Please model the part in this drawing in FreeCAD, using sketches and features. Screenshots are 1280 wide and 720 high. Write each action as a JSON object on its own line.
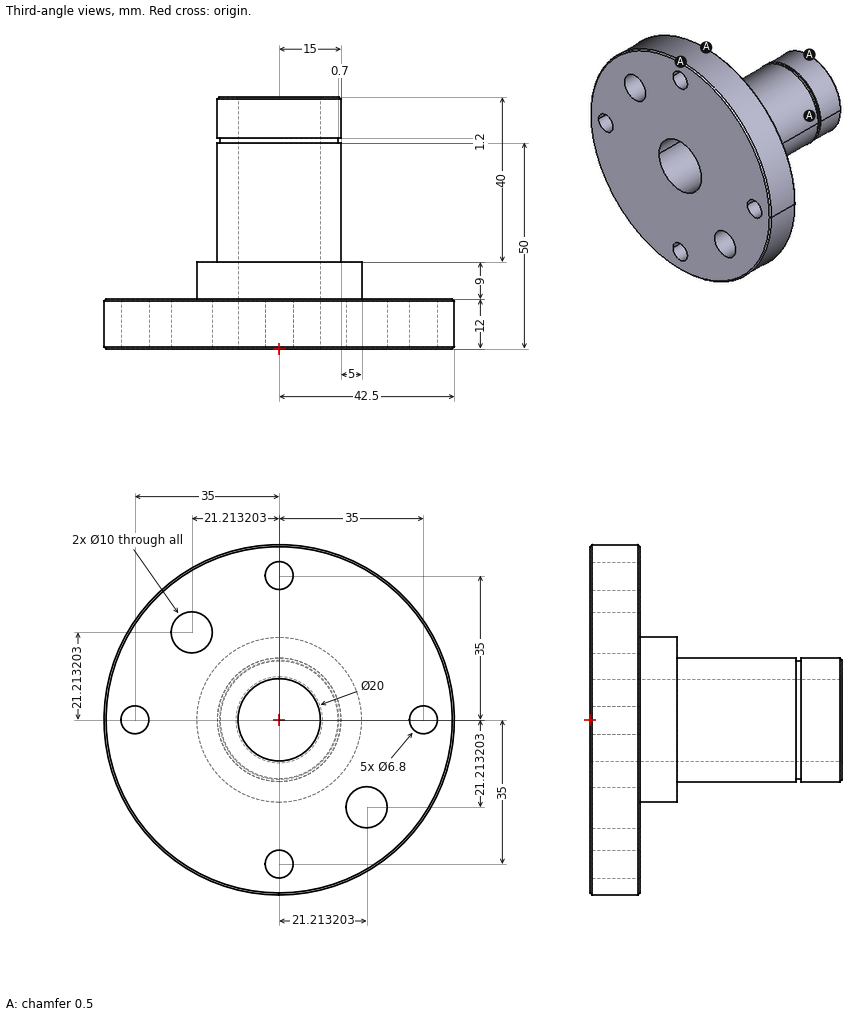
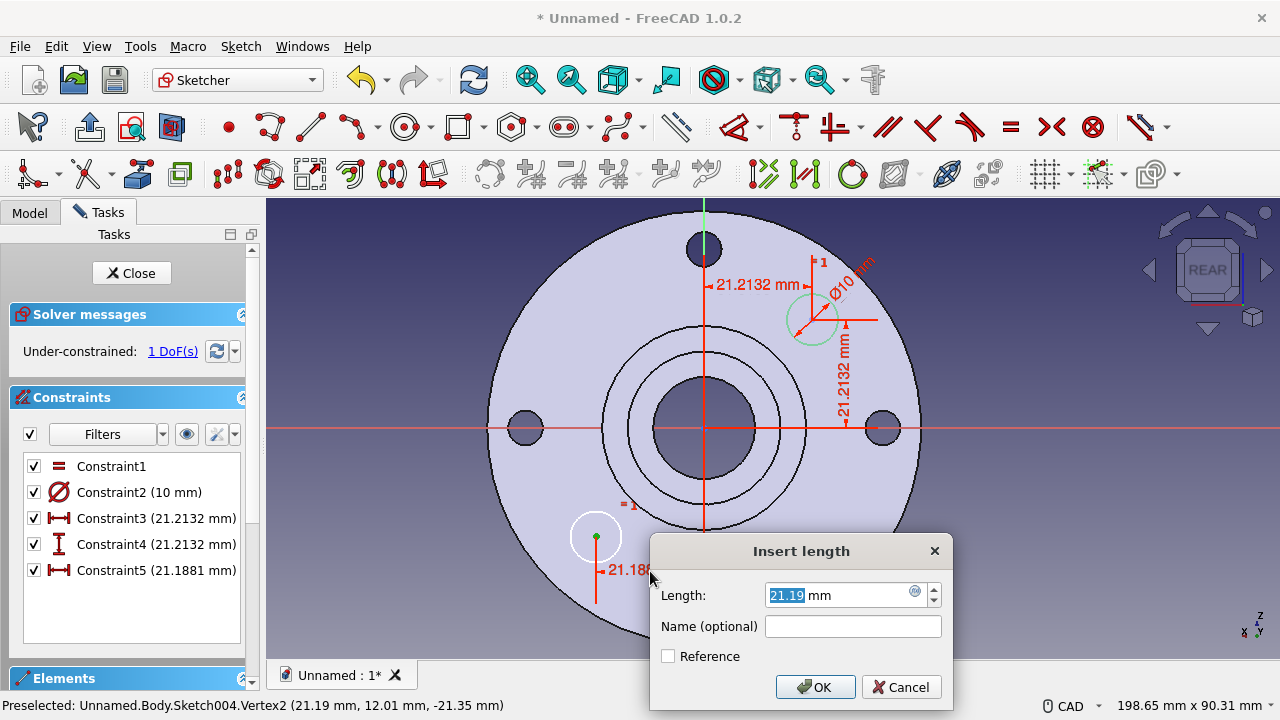
{"action": "type", "text": "21.213203"}
{"action": "key", "text": "Return"}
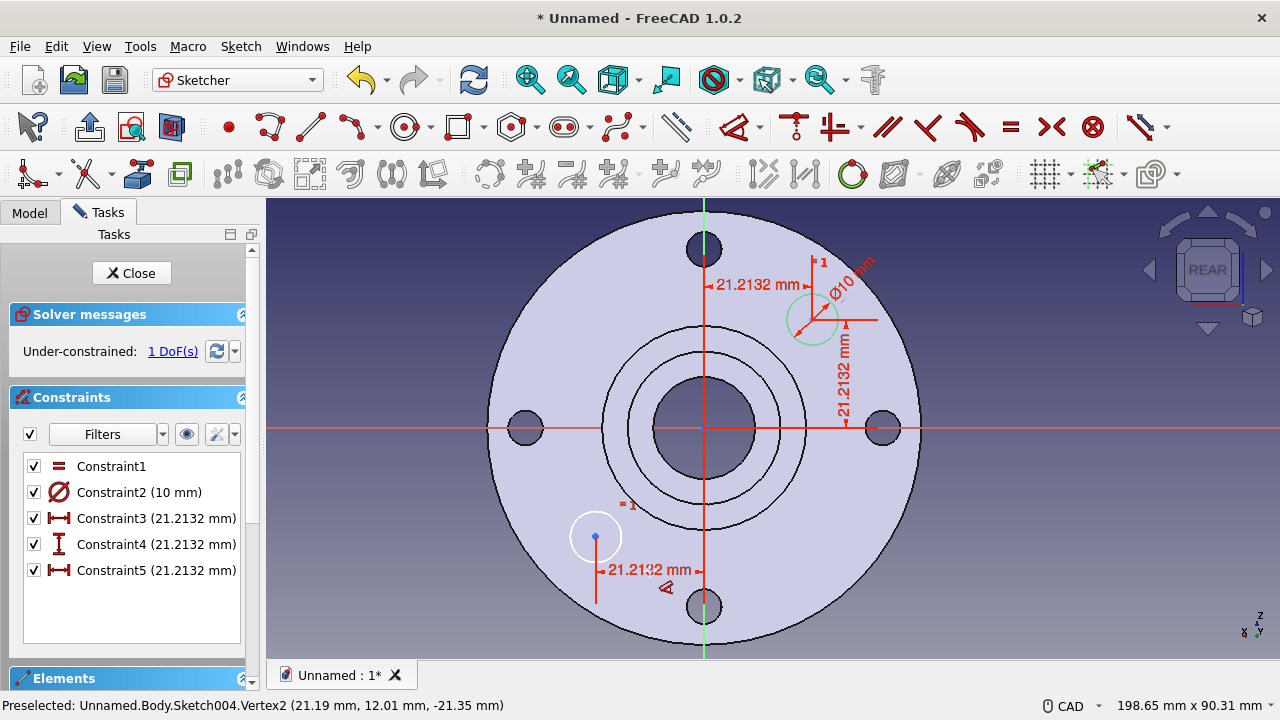
{"action": "left_click", "coordinate": [596, 537]}
{"action": "left_click", "coordinate": [562, 483]}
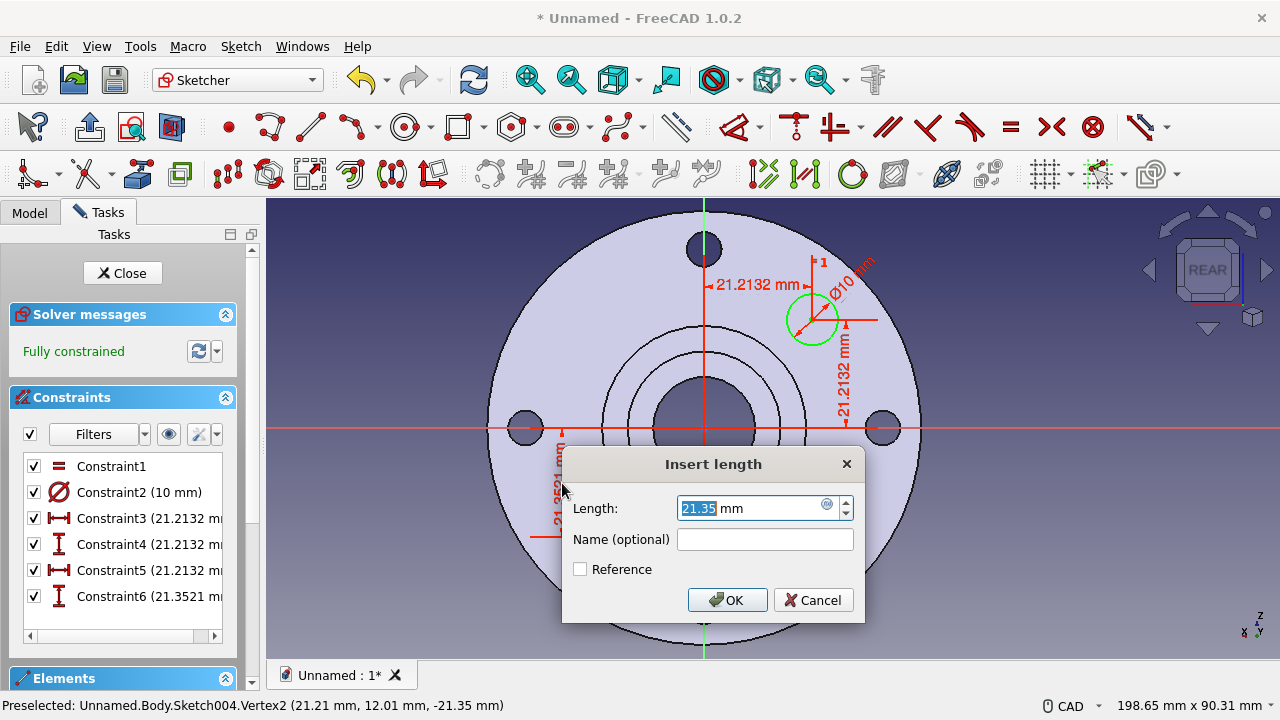
{"action": "type", "text": "21.213203"}
{"action": "key", "text": "Return"}
{"action": "key", "text": "Escape"}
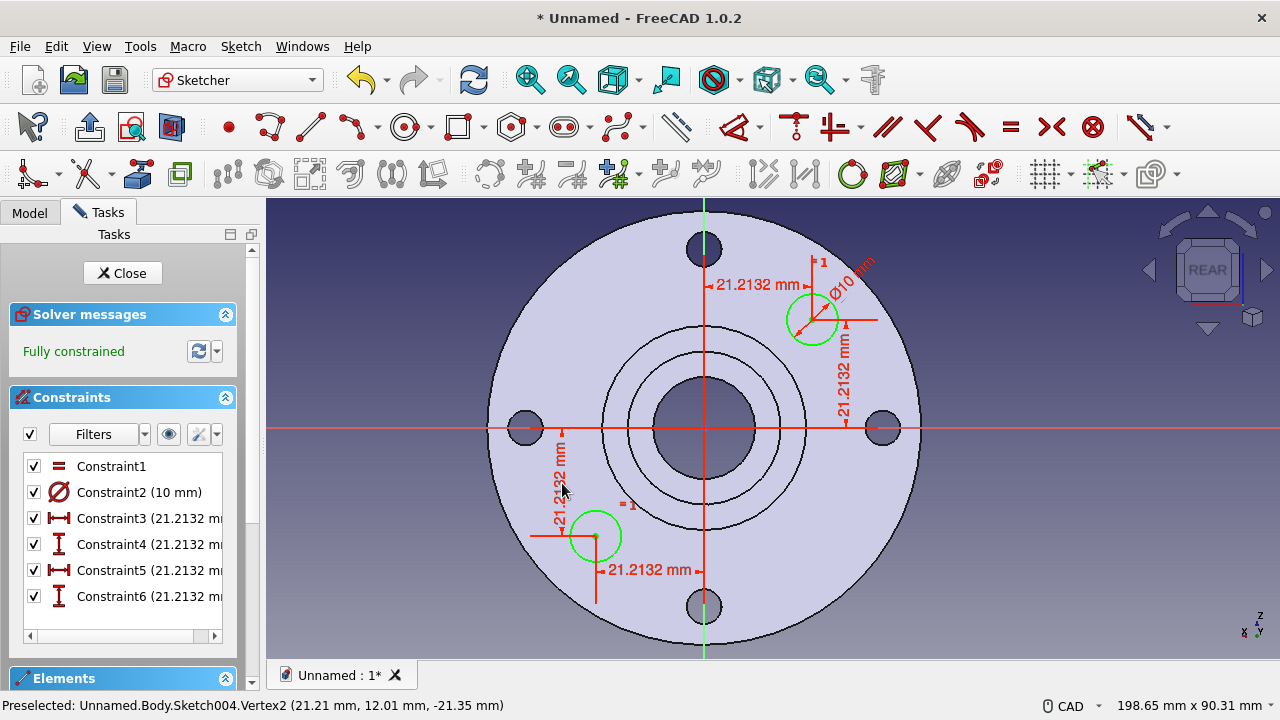
{"action": "left_click", "coordinate": [123, 273]}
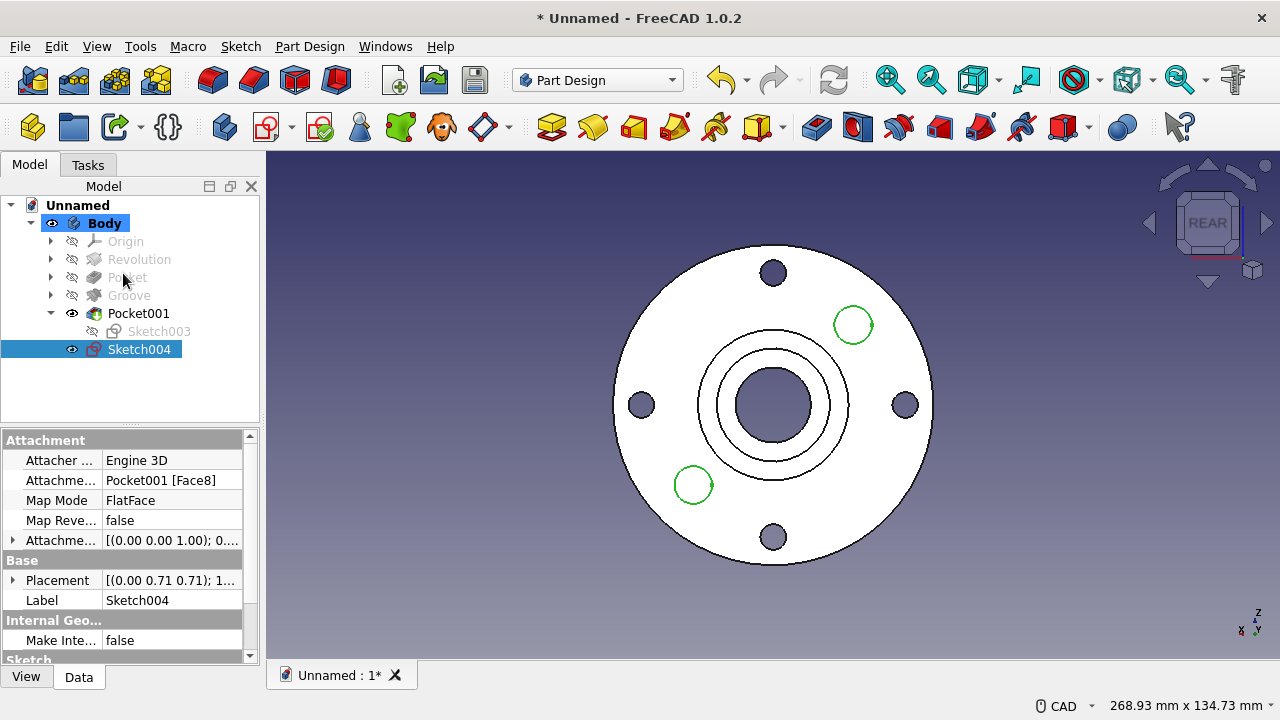
{"action": "left_click", "coordinate": [858, 128]}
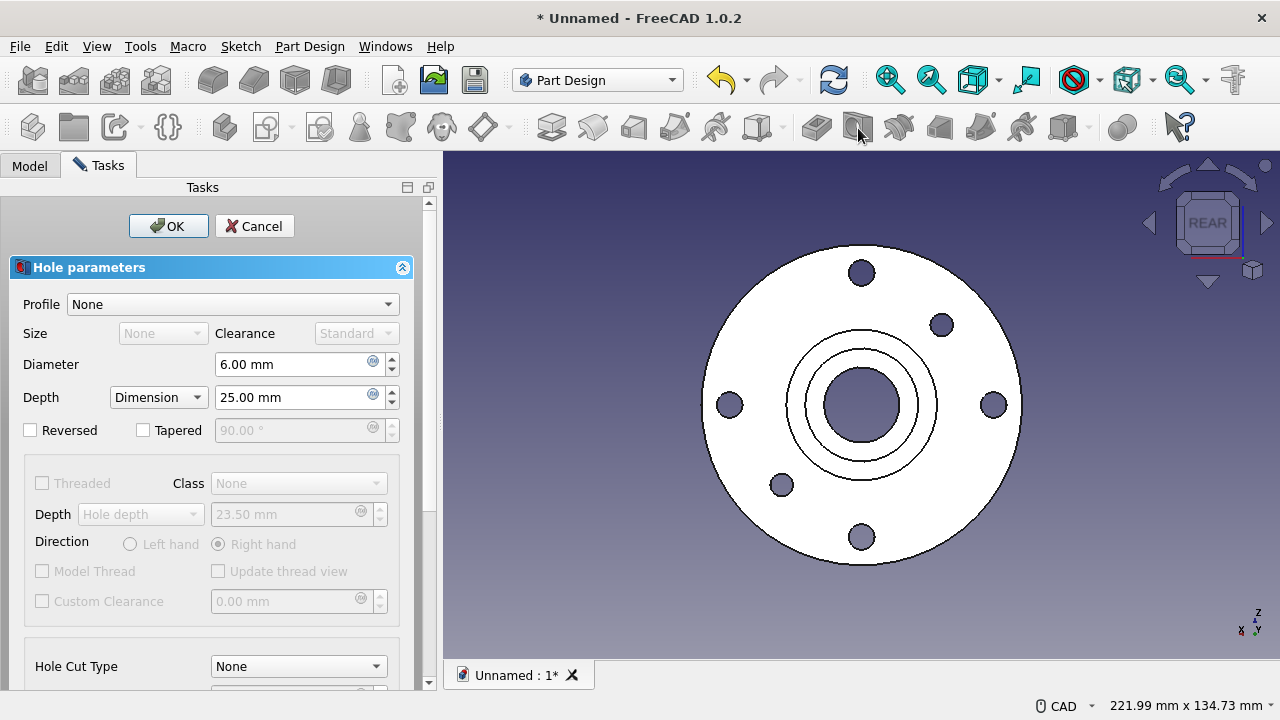
{"action": "triple_click", "coordinate": [300, 364]}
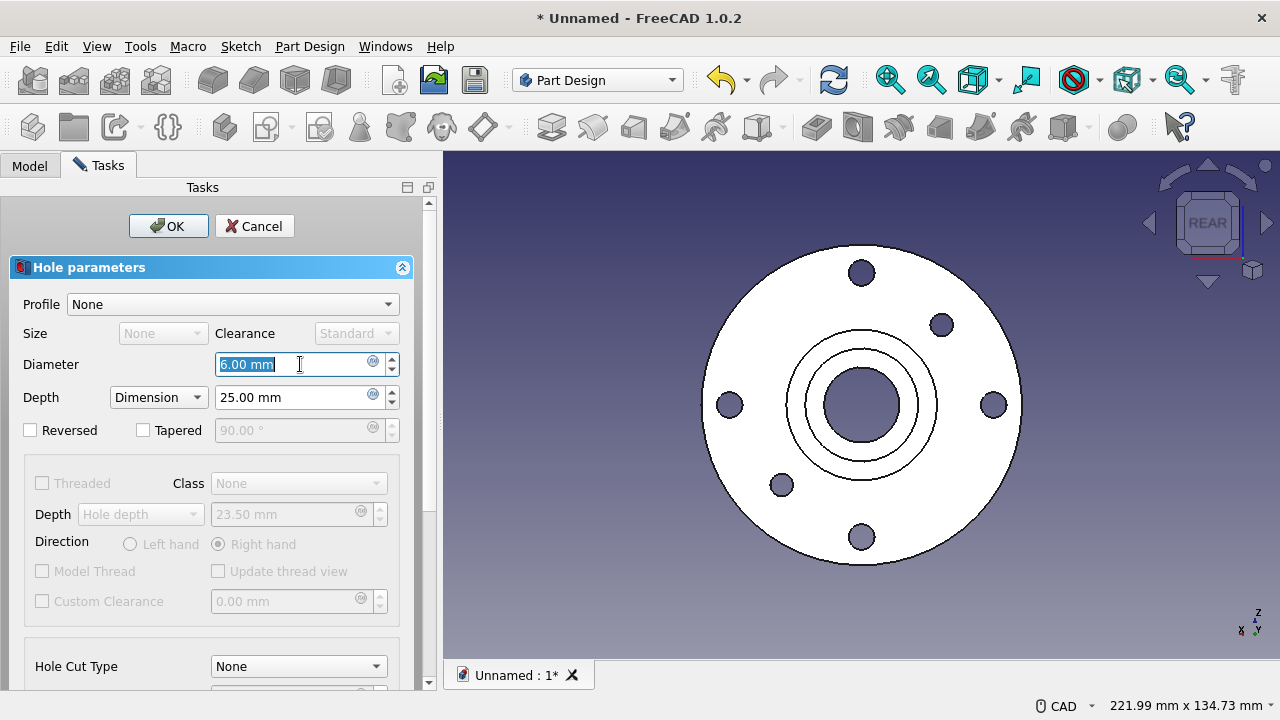
{"action": "type", "text": "10"}
{"action": "key", "text": "Tab"}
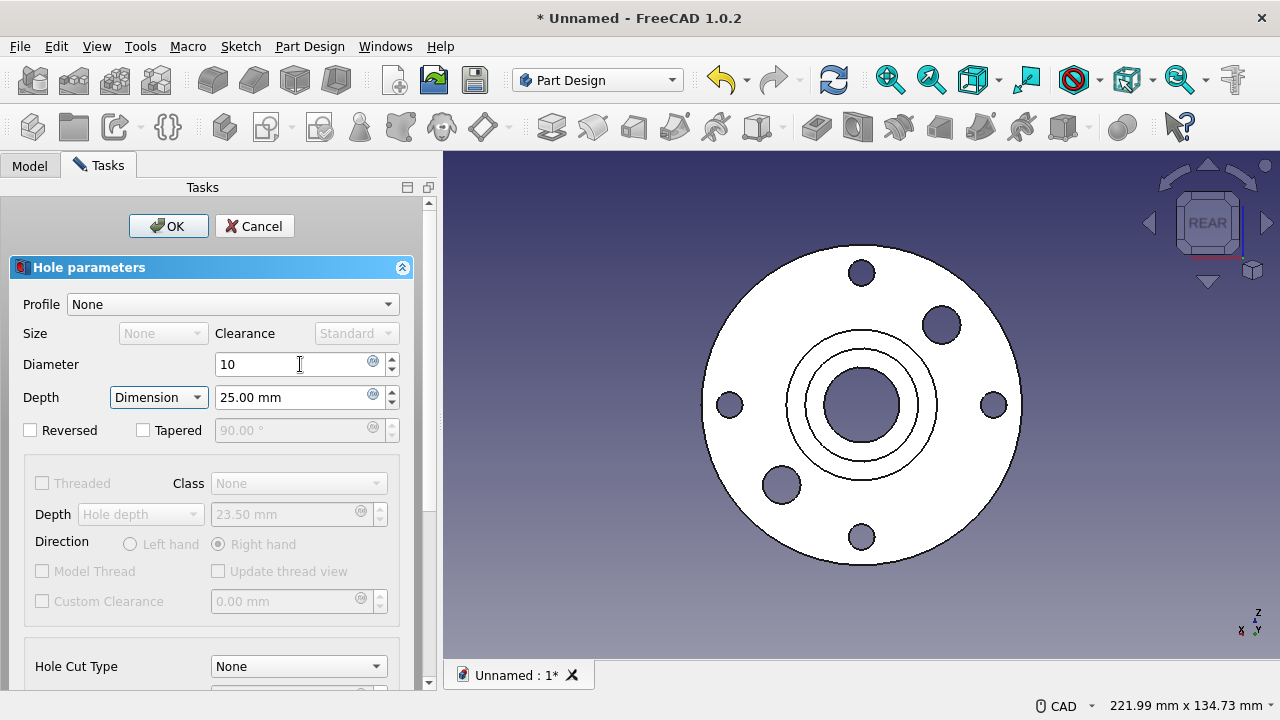
{"action": "left_click", "coordinate": [160, 398]}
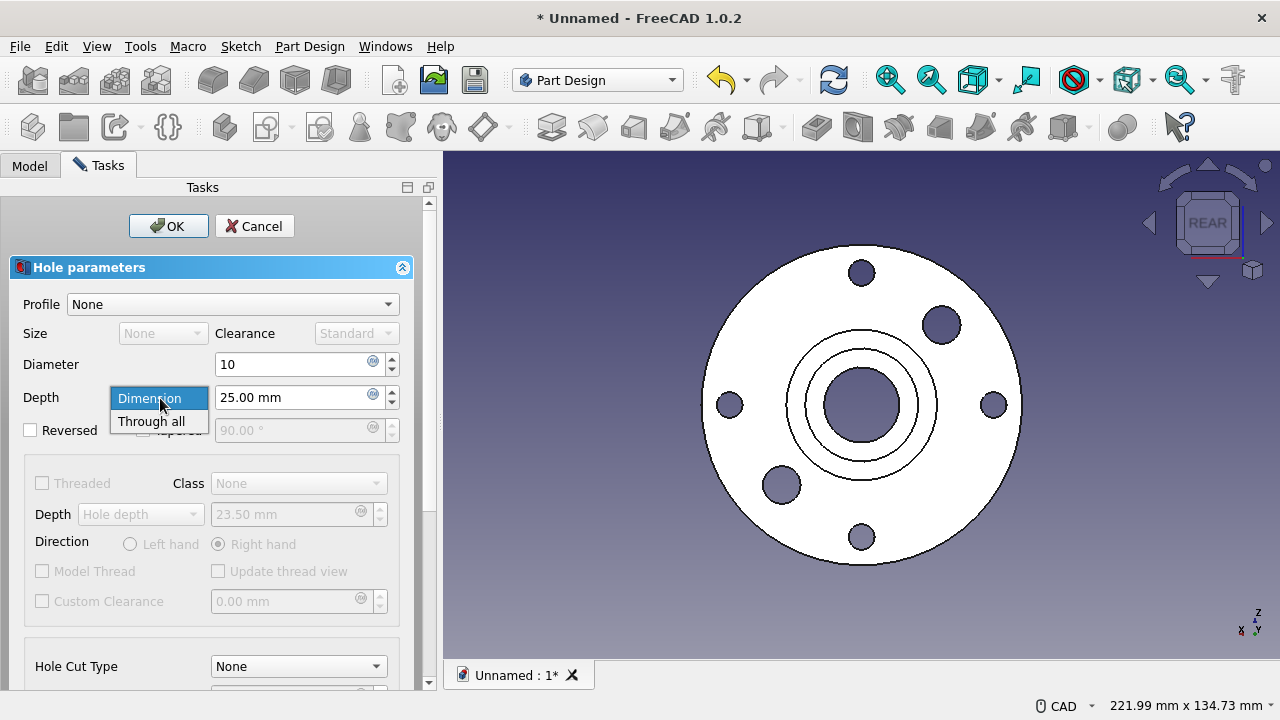
{"action": "left_click", "coordinate": [158, 422]}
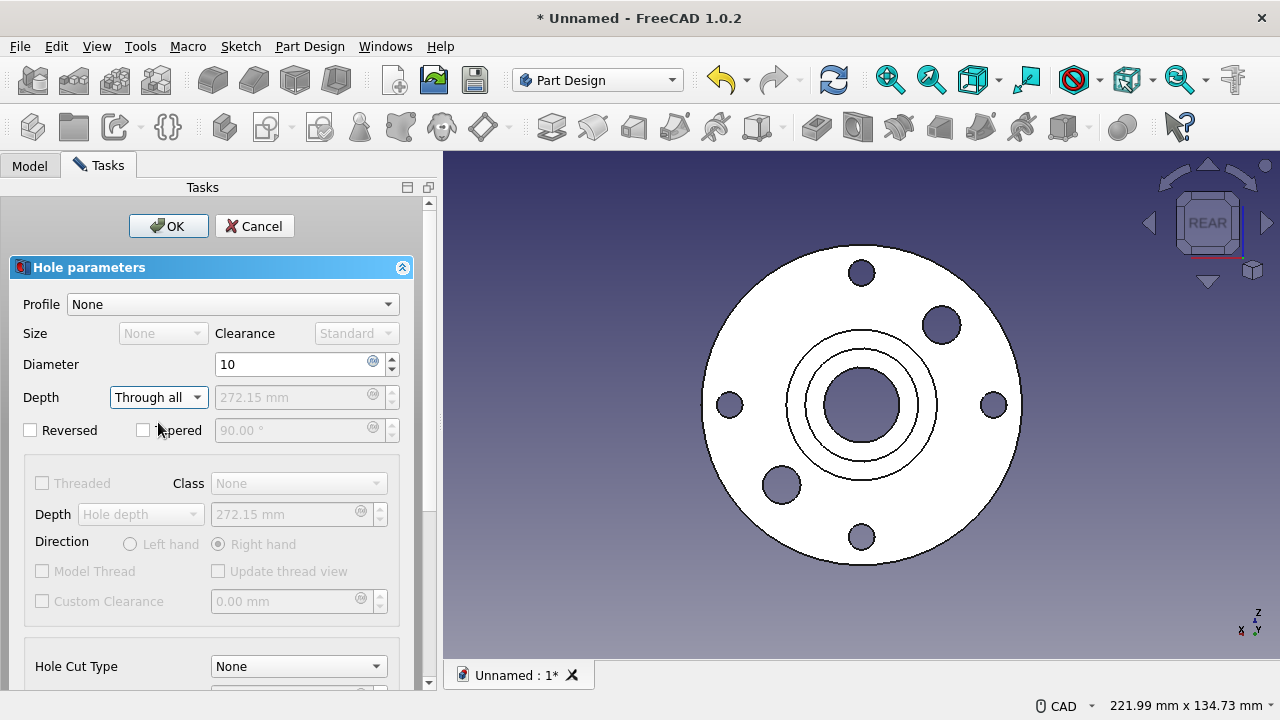
{"action": "left_click", "coordinate": [169, 226]}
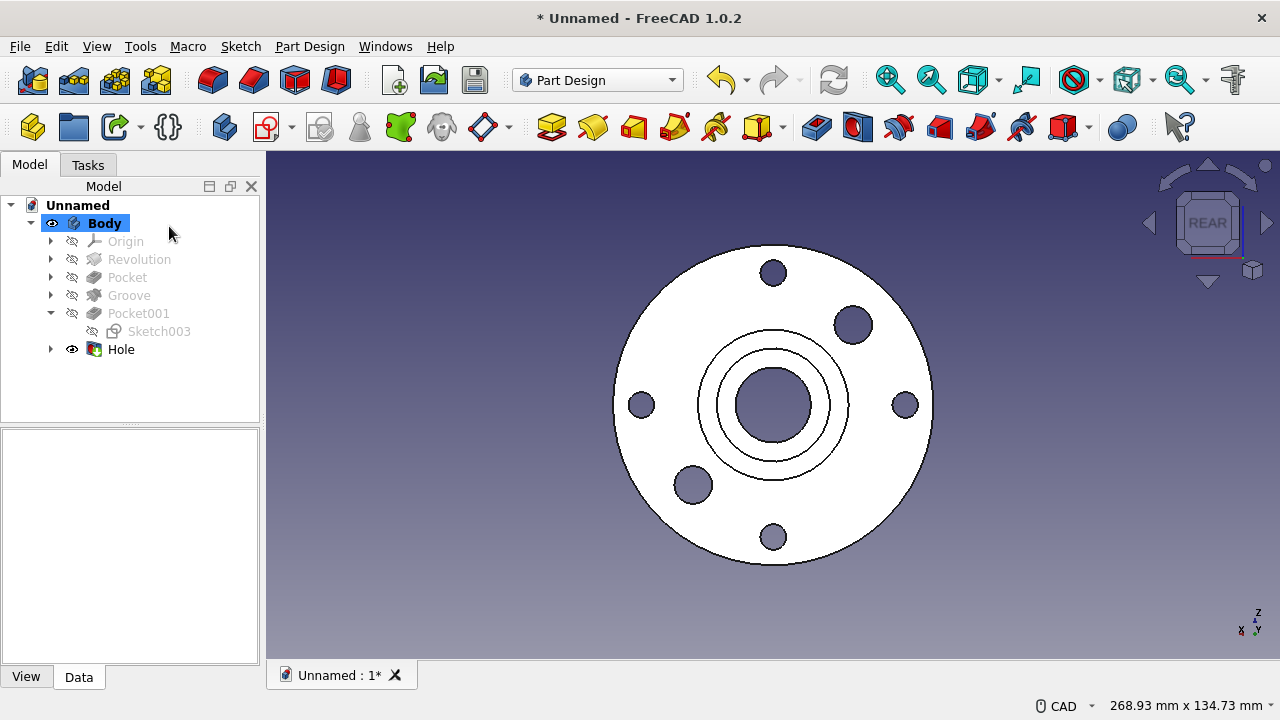
{"action": "left_click", "coordinate": [736, 404]}